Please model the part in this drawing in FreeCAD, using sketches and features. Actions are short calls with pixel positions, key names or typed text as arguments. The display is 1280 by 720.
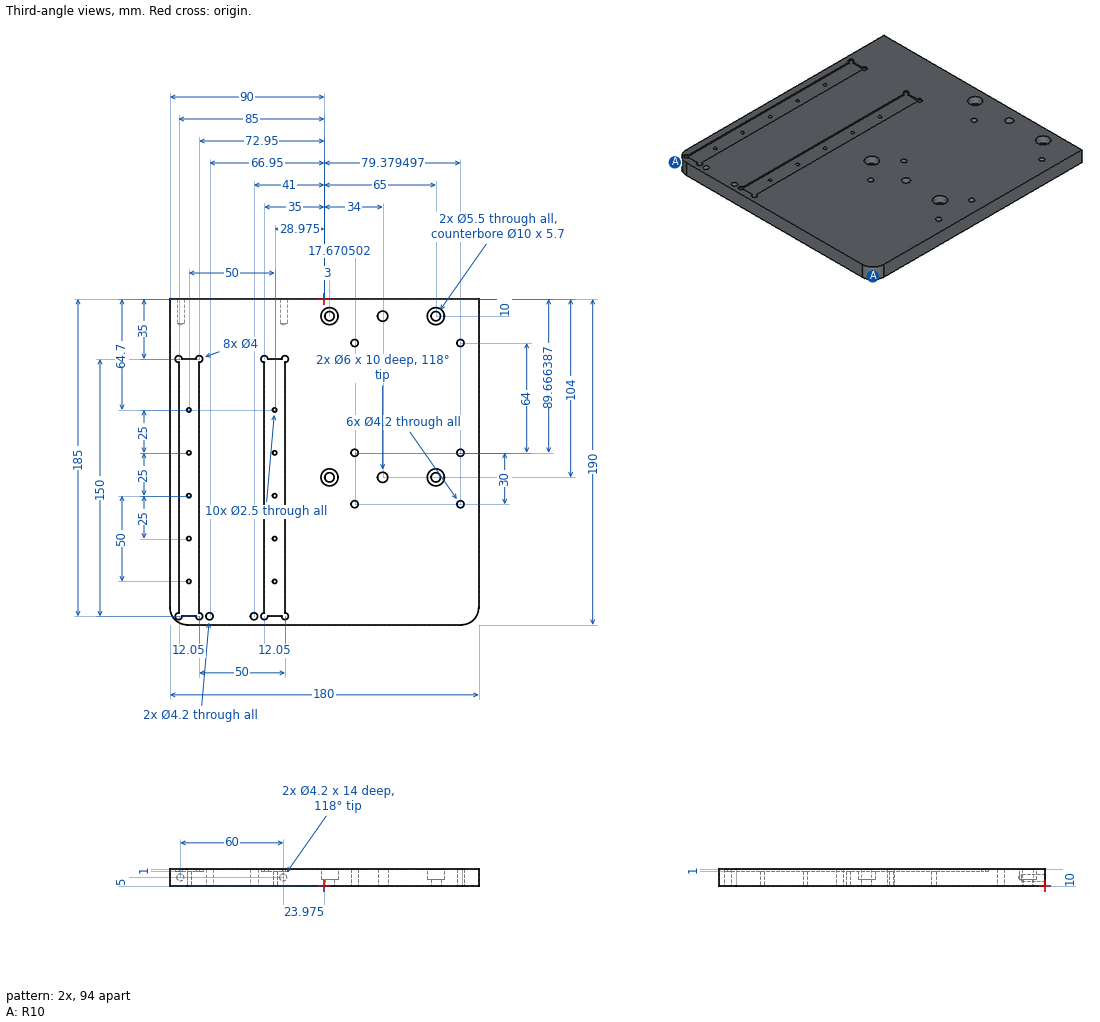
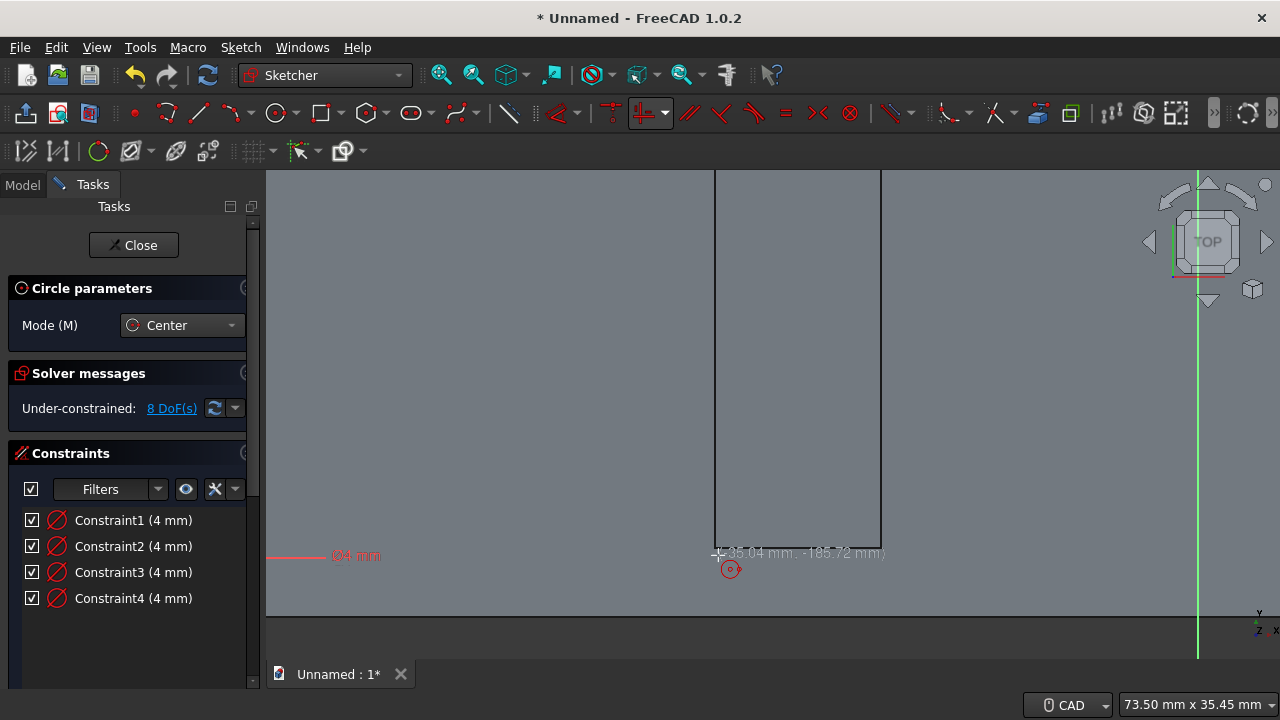
scroll(718, 555, down, 11)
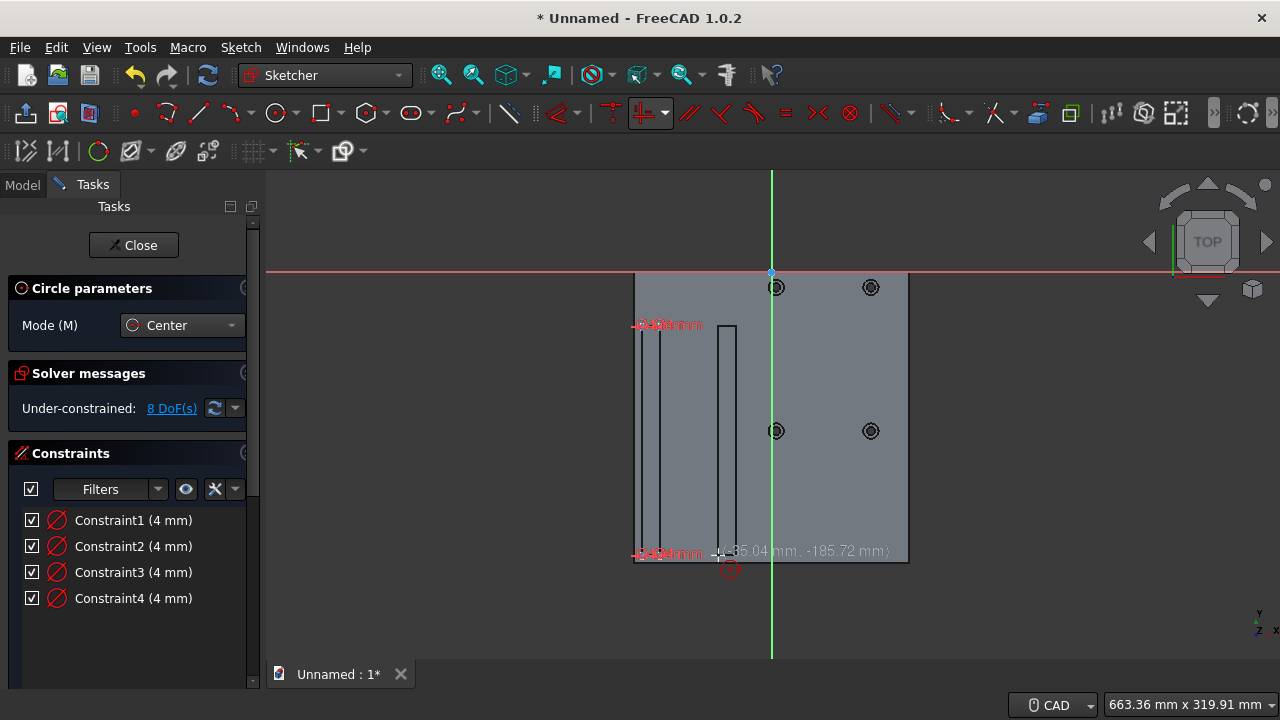
click(718, 555)
move(720, 553)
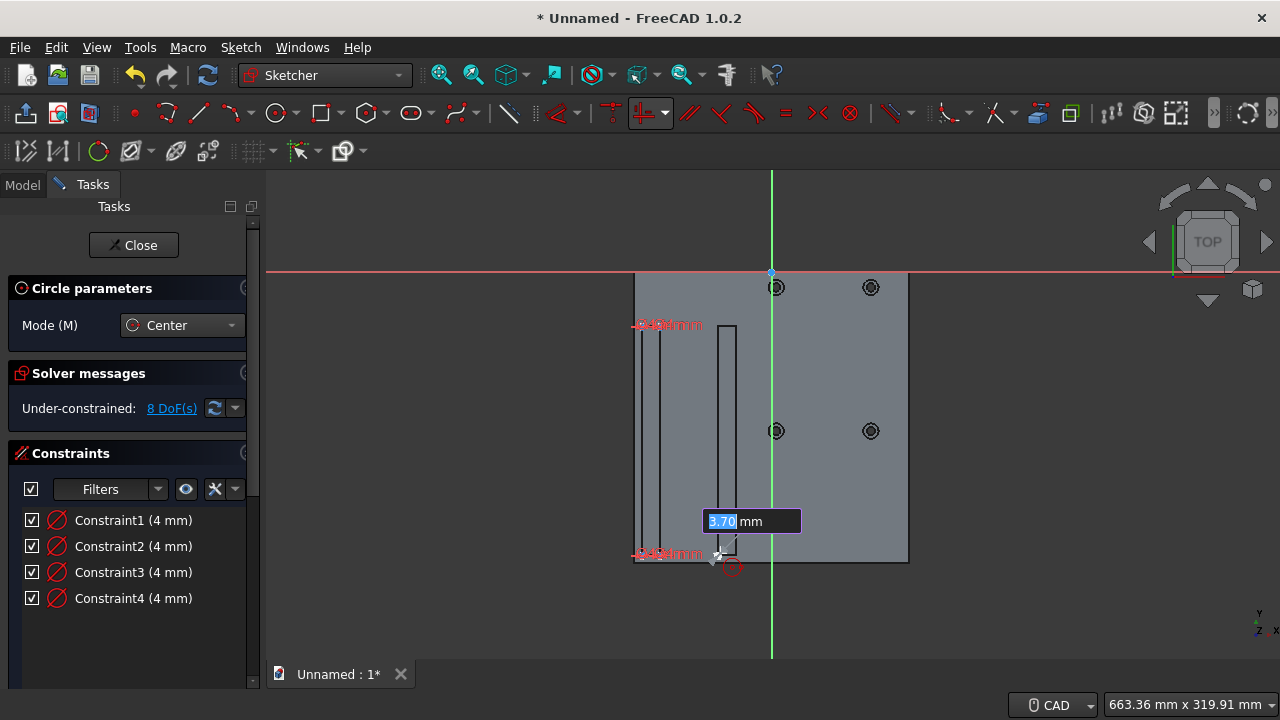
text(4)
key(Return)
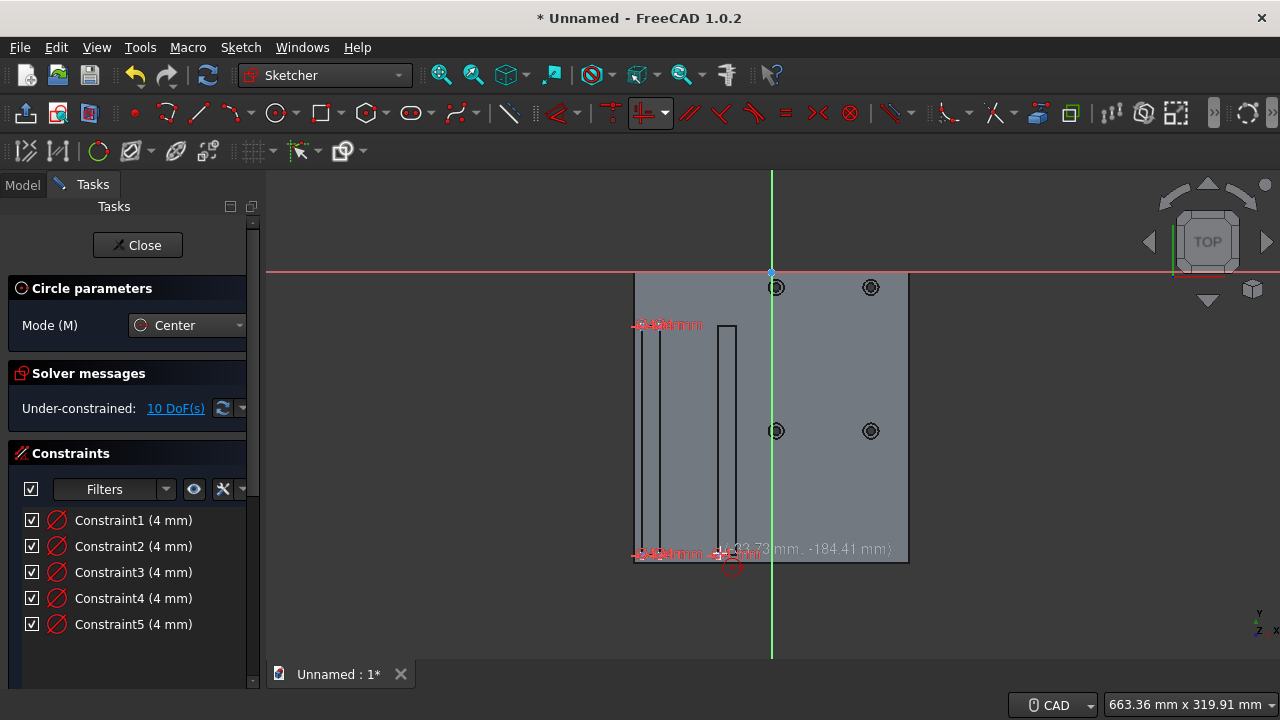
scroll(736, 555, up, 11)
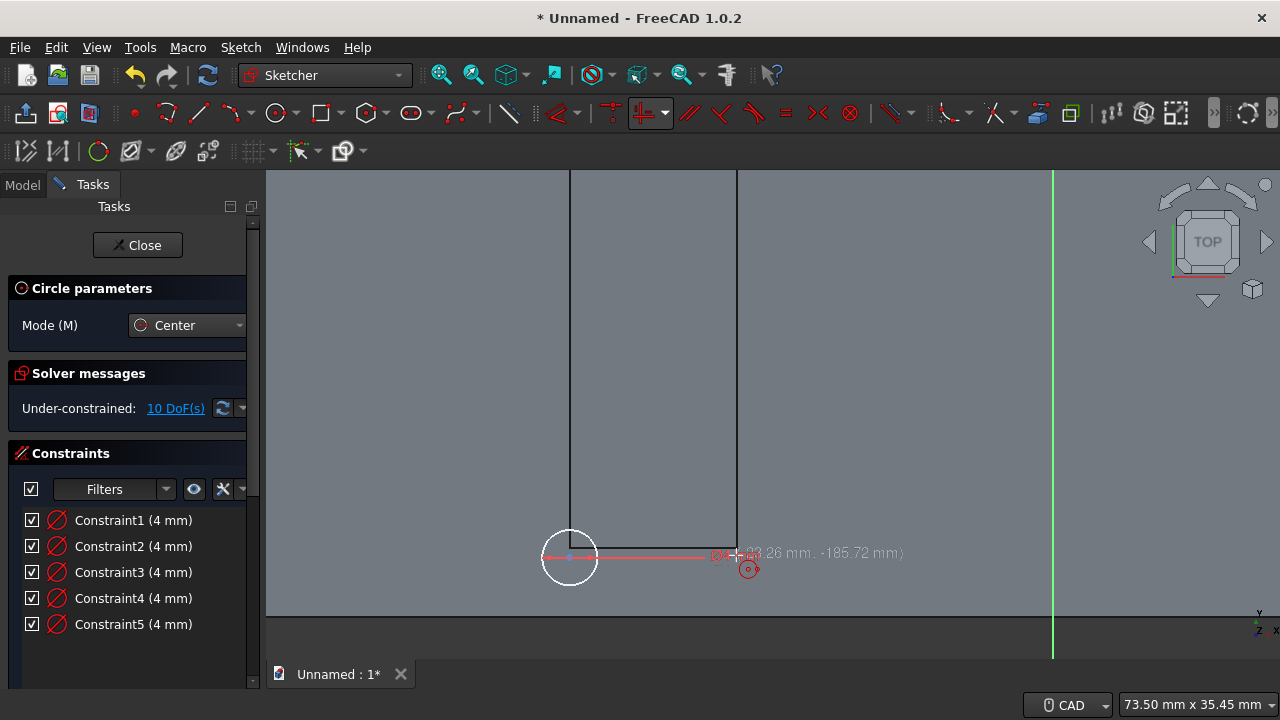
scroll(736, 555, down, 11)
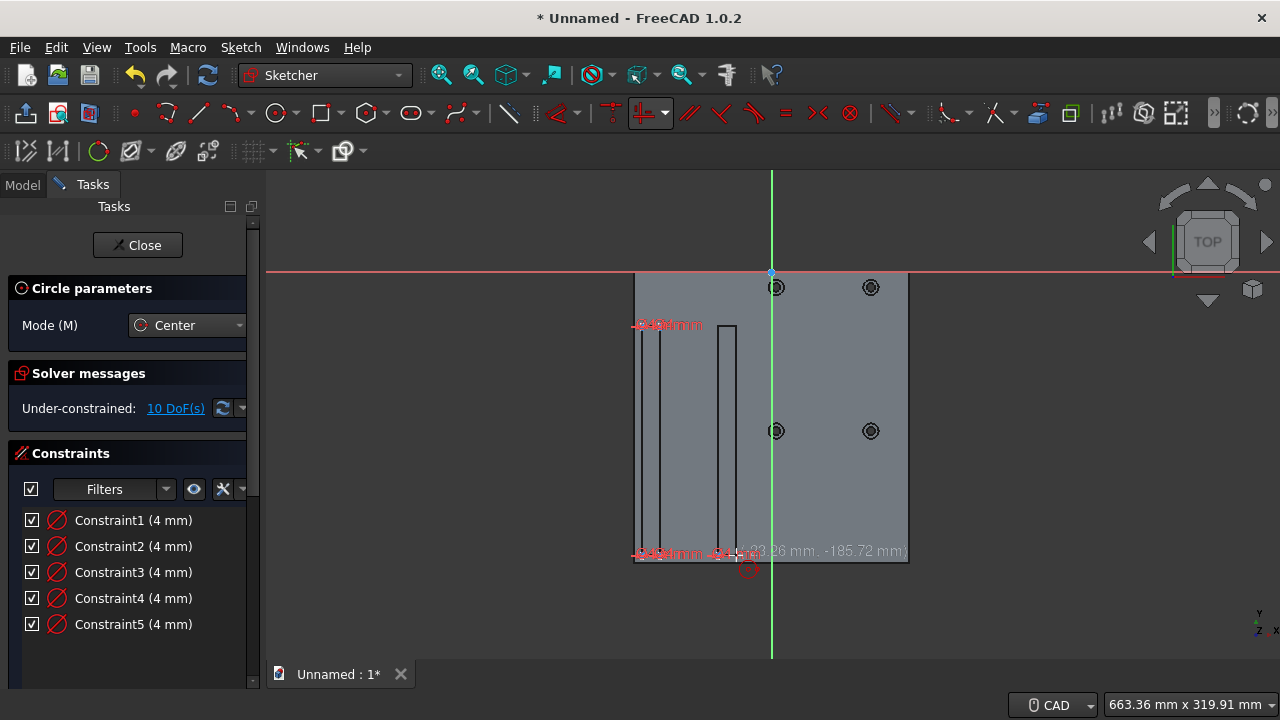
click(736, 555)
move(739, 553)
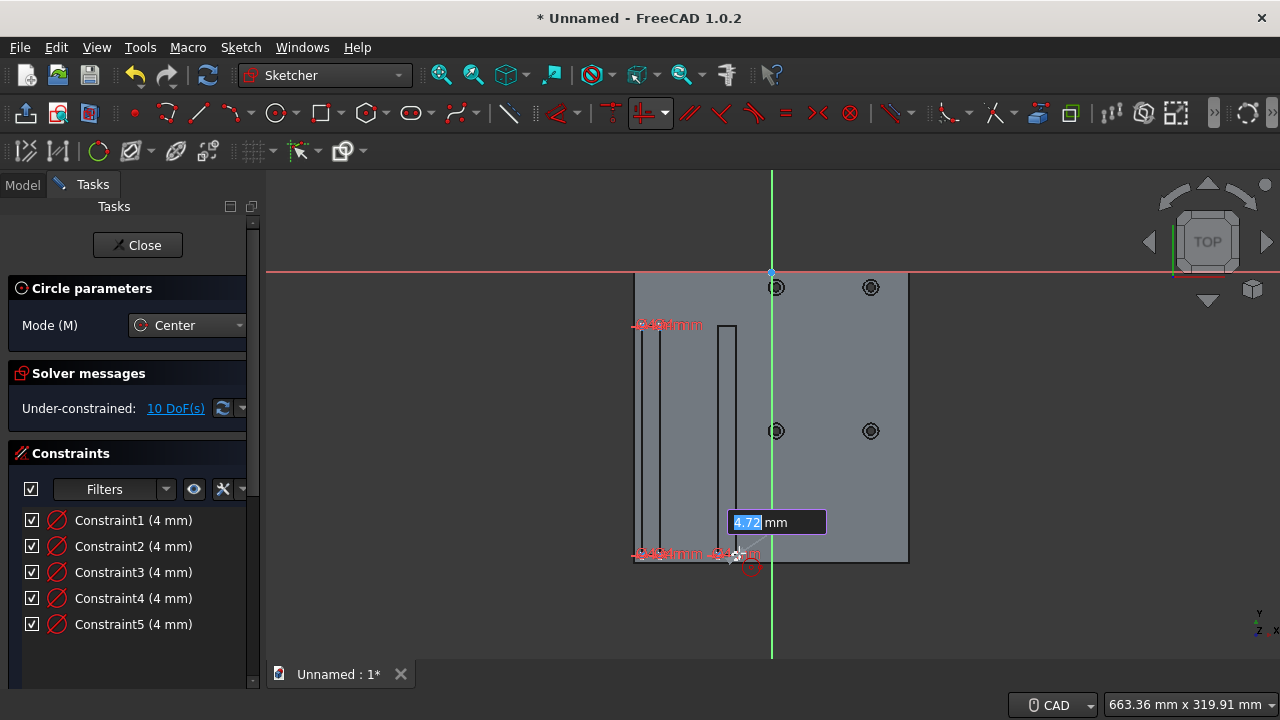
text(4)
key(Return)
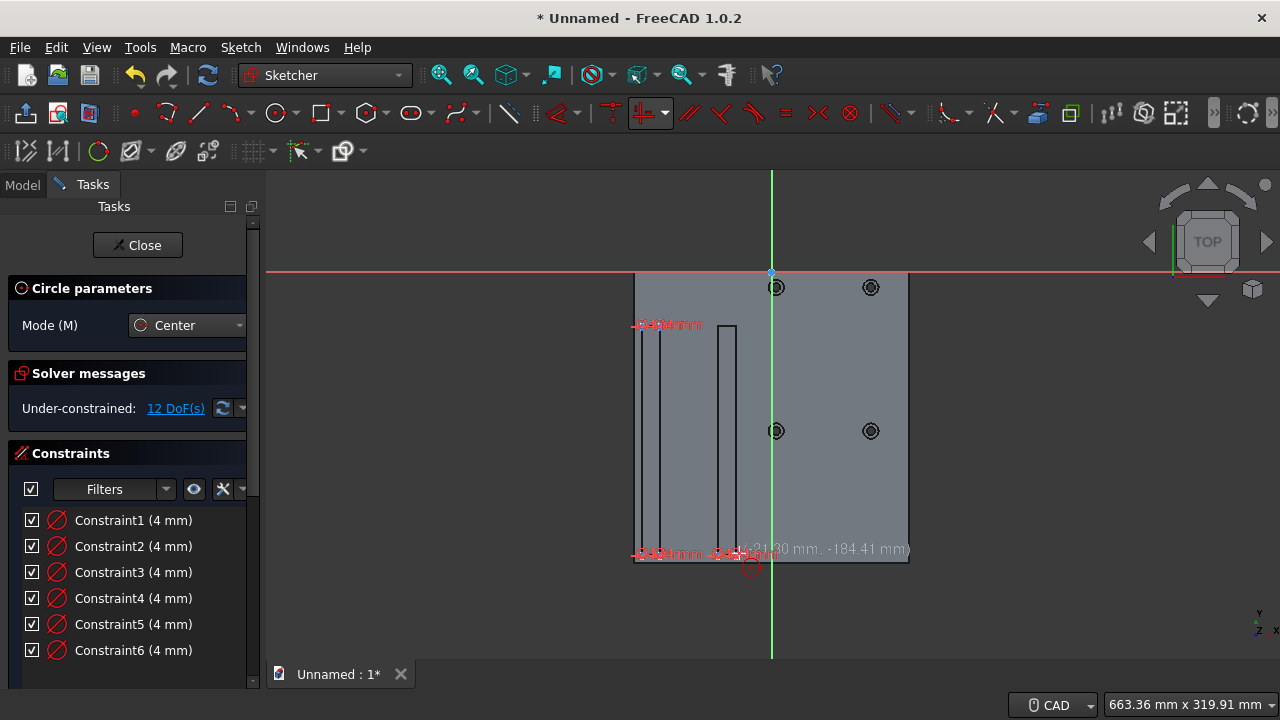
scroll(718, 326, up, 11)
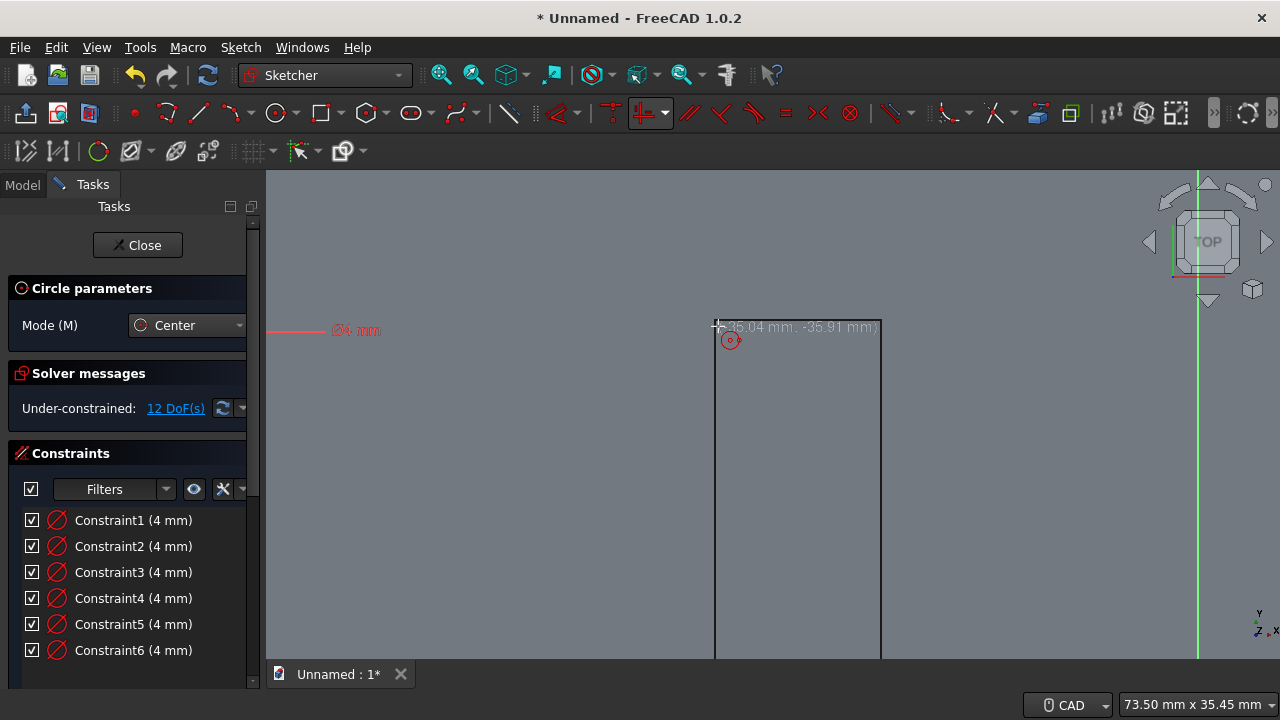
scroll(718, 326, down, 11)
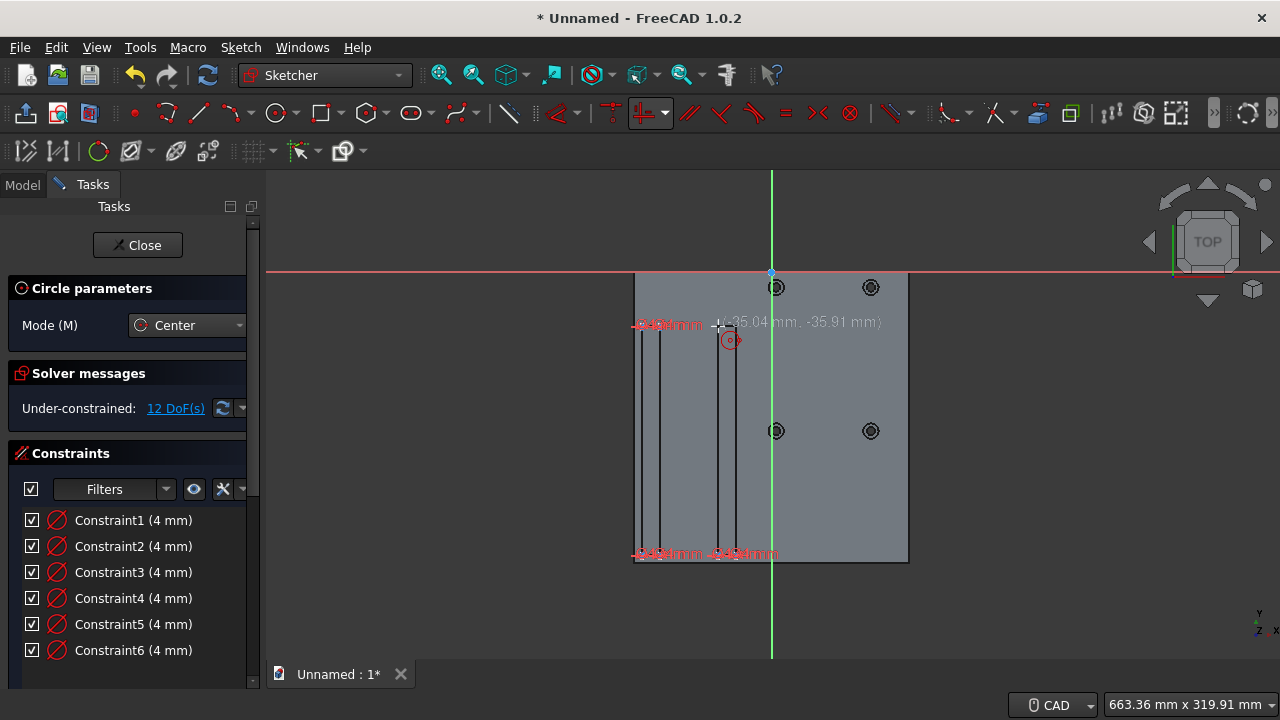
click(718, 326)
move(720, 323)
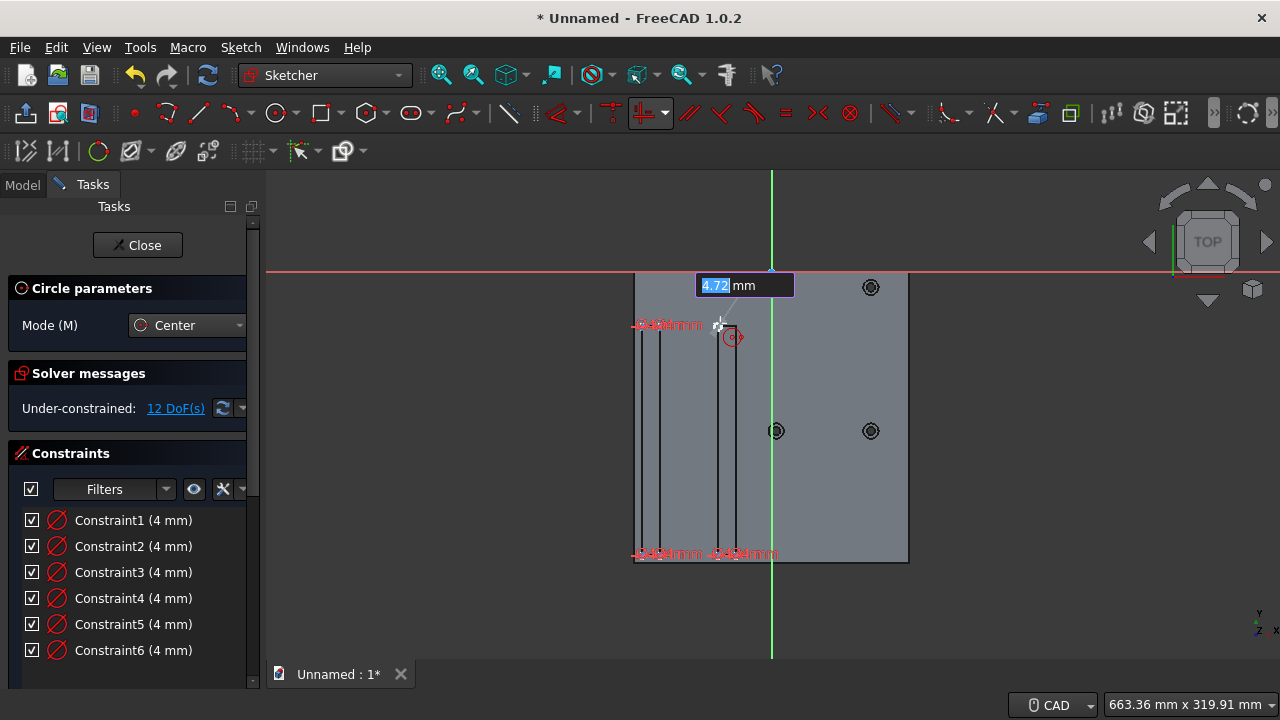
text(4)
key(Return)